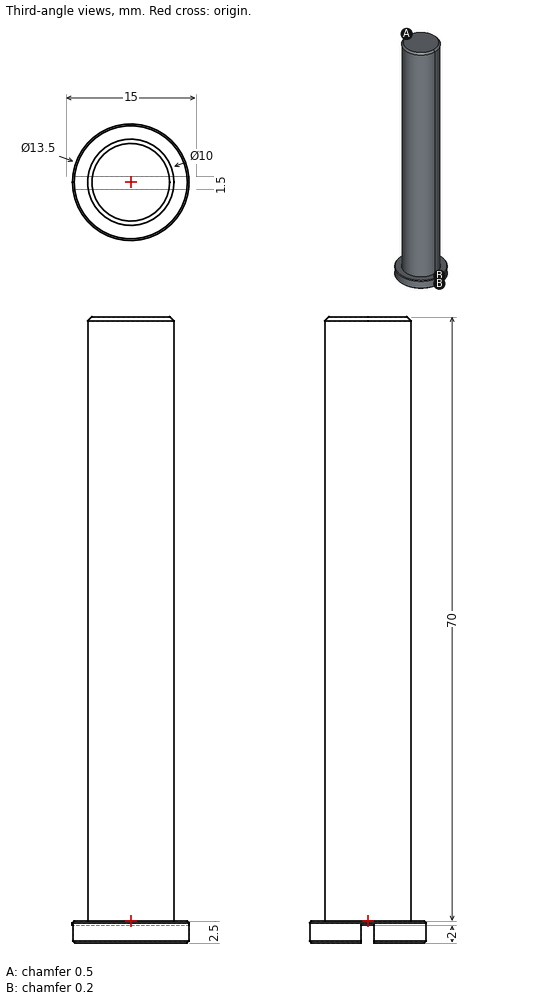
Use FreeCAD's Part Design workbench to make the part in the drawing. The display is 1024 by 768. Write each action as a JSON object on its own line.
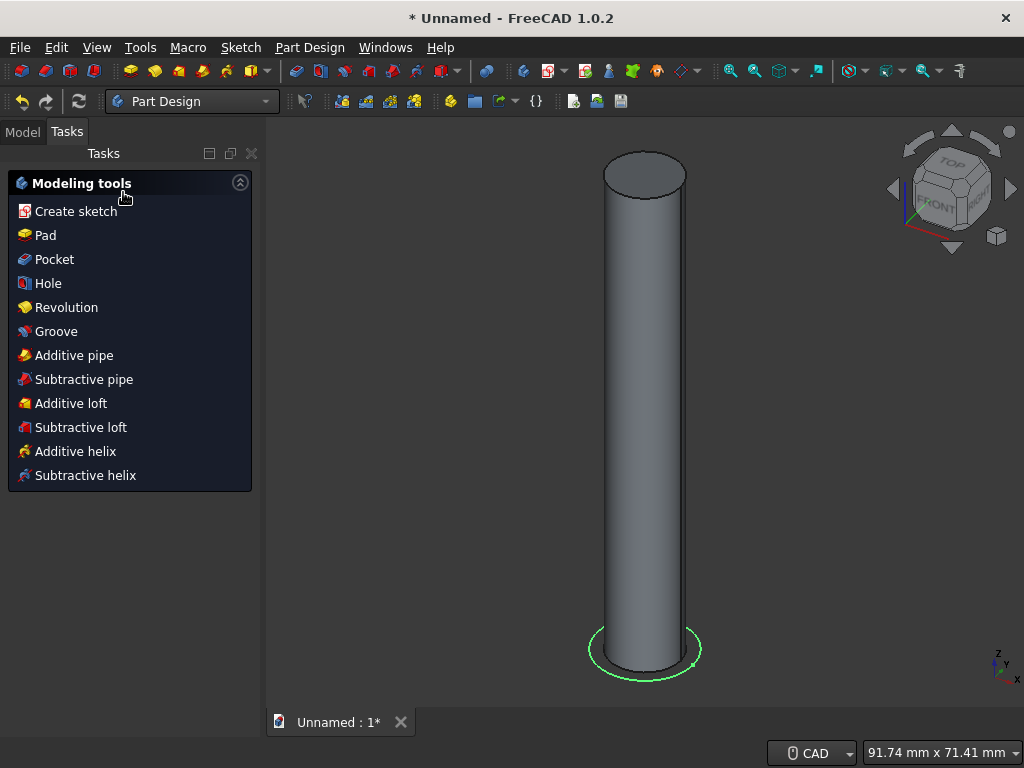
{"action": "left_click", "coordinate": [132, 72]}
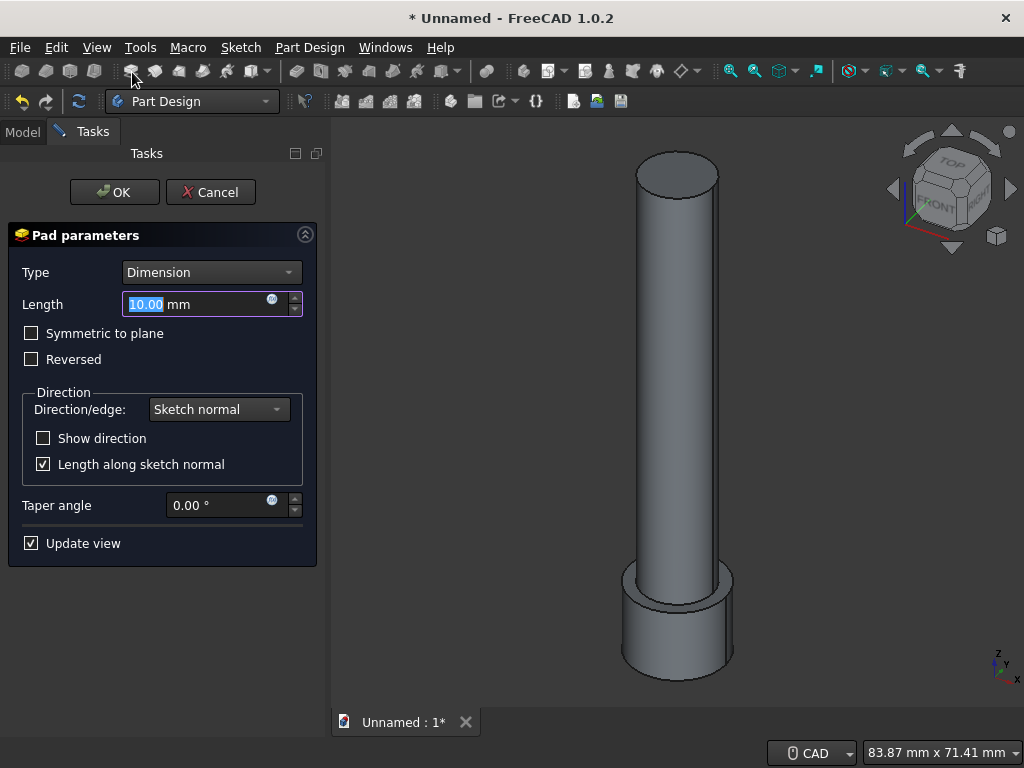
{"action": "type", "text": "2.5"}
{"action": "key", "text": "Tab"}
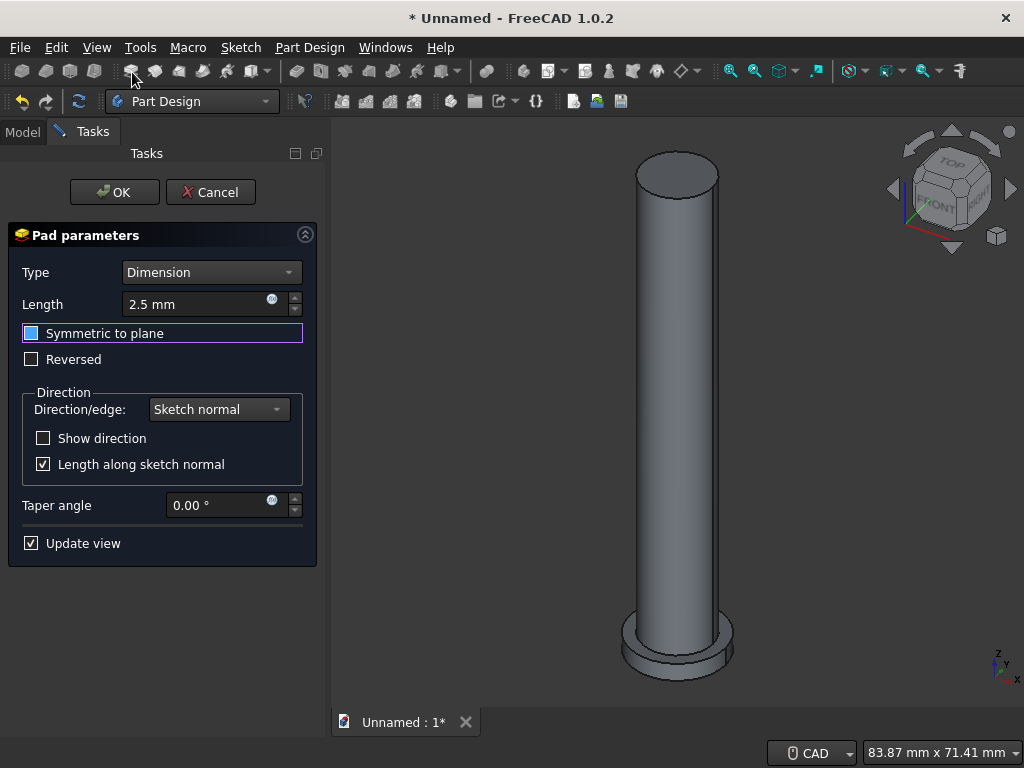
{"action": "left_click", "coordinate": [30, 359]}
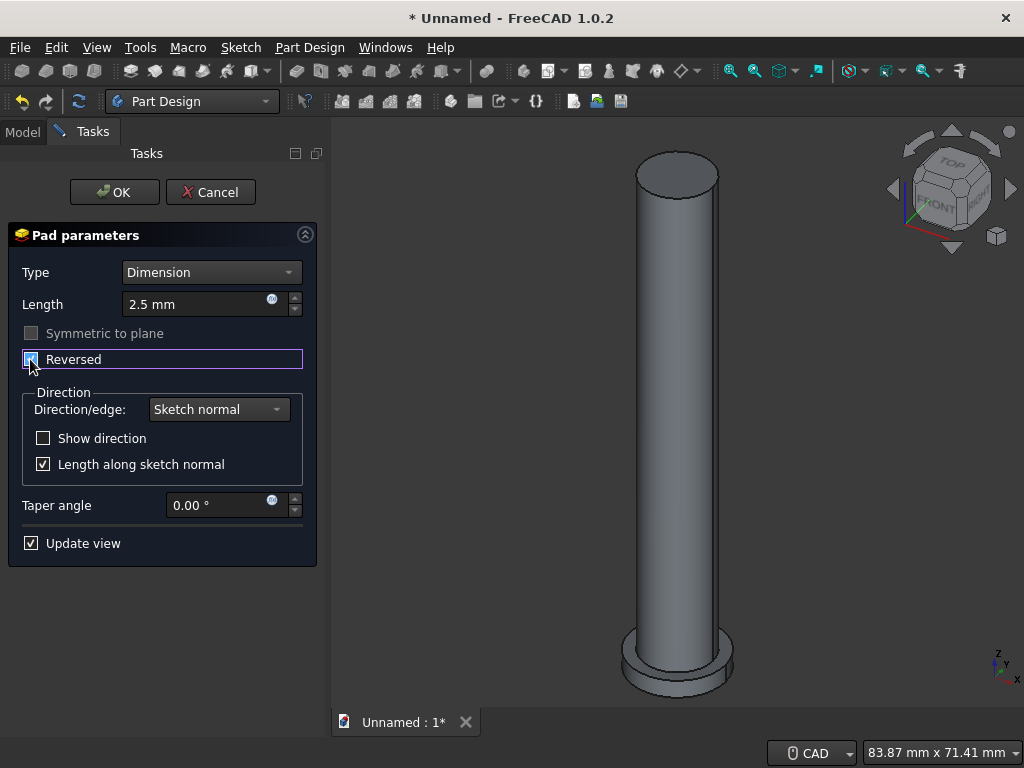
{"action": "left_click", "coordinate": [115, 192]}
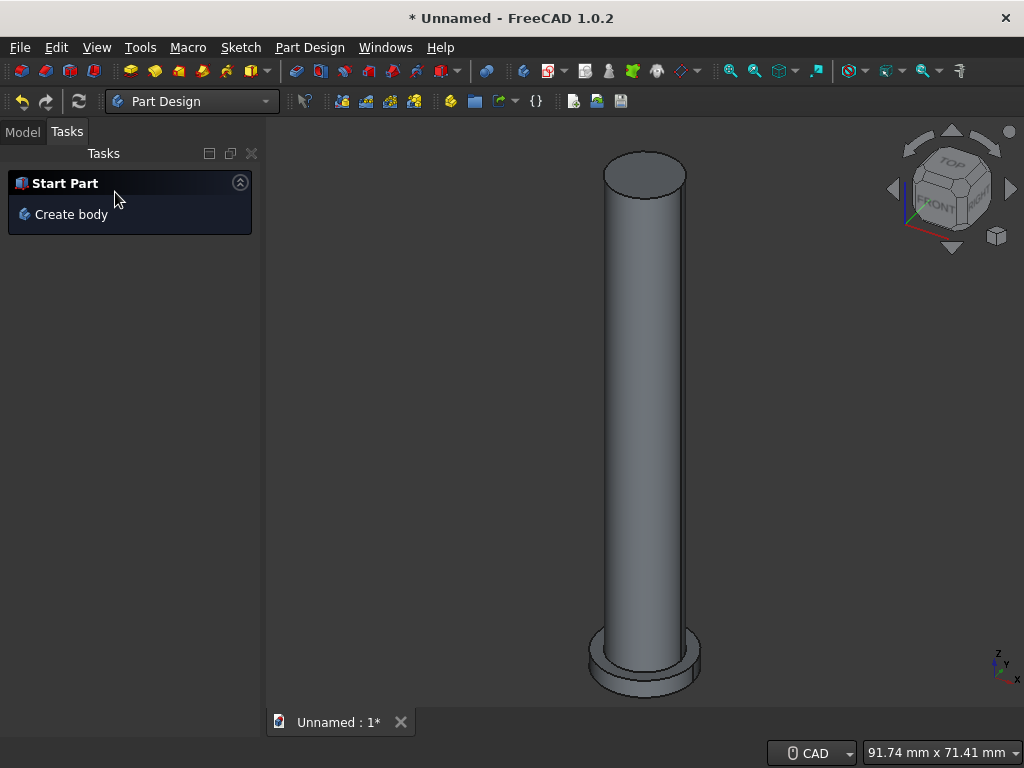
{"action": "left_click", "coordinate": [732, 72]}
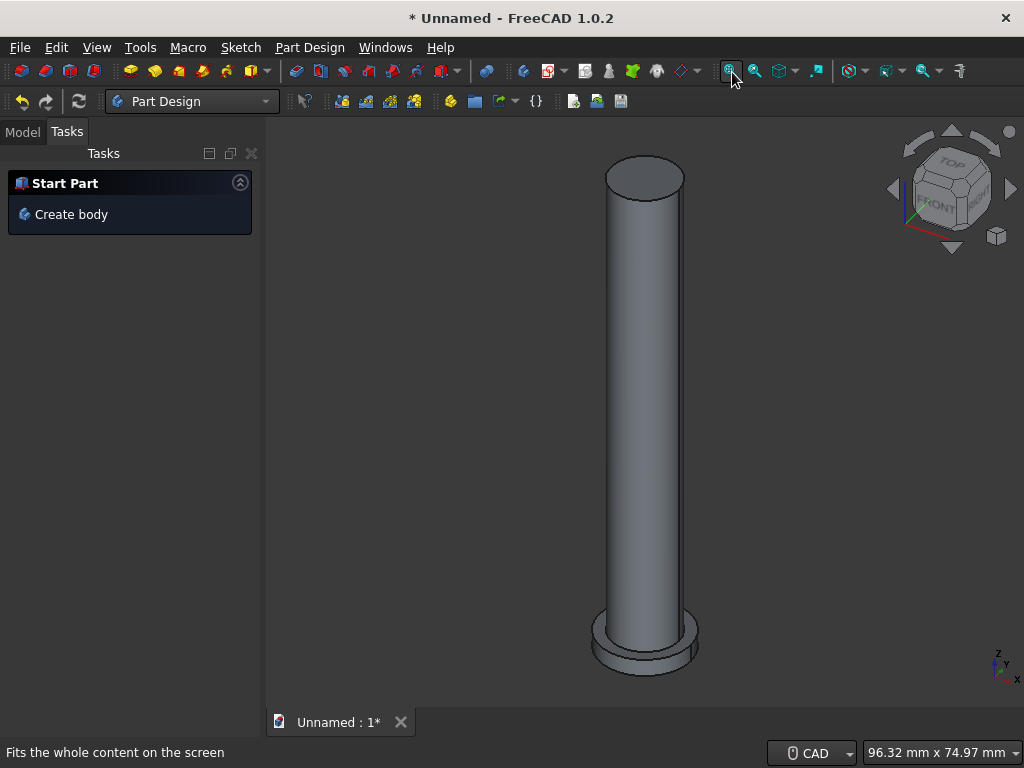
{"action": "left_click", "coordinate": [611, 166]}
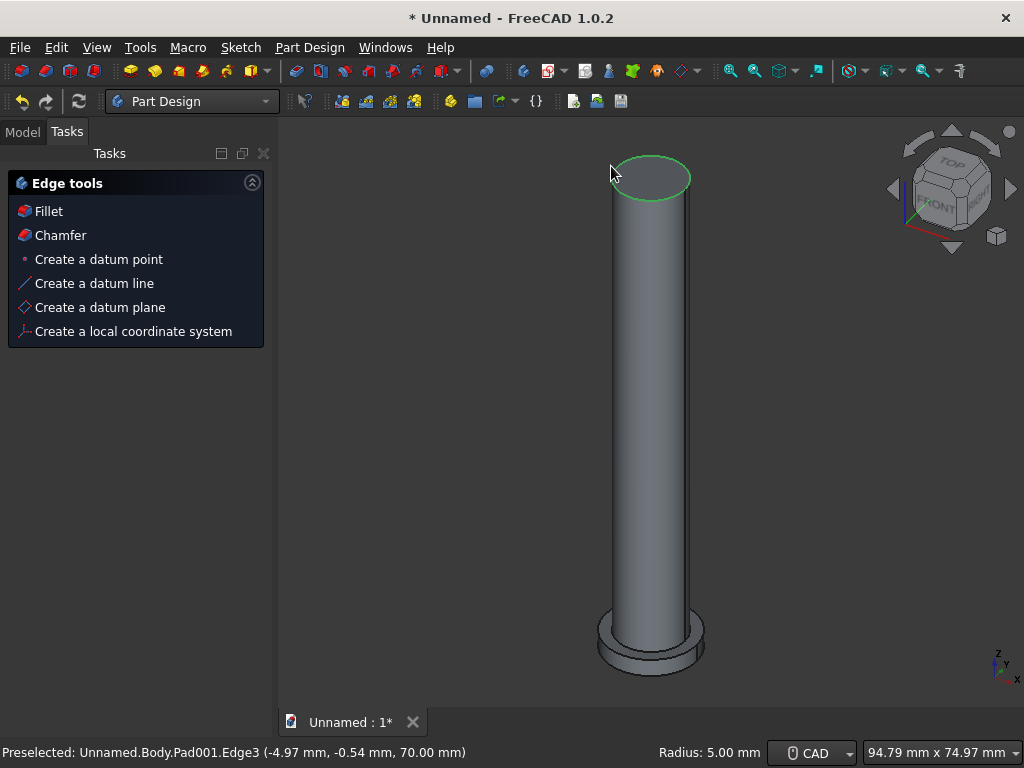
{"action": "left_click", "coordinate": [46, 72]}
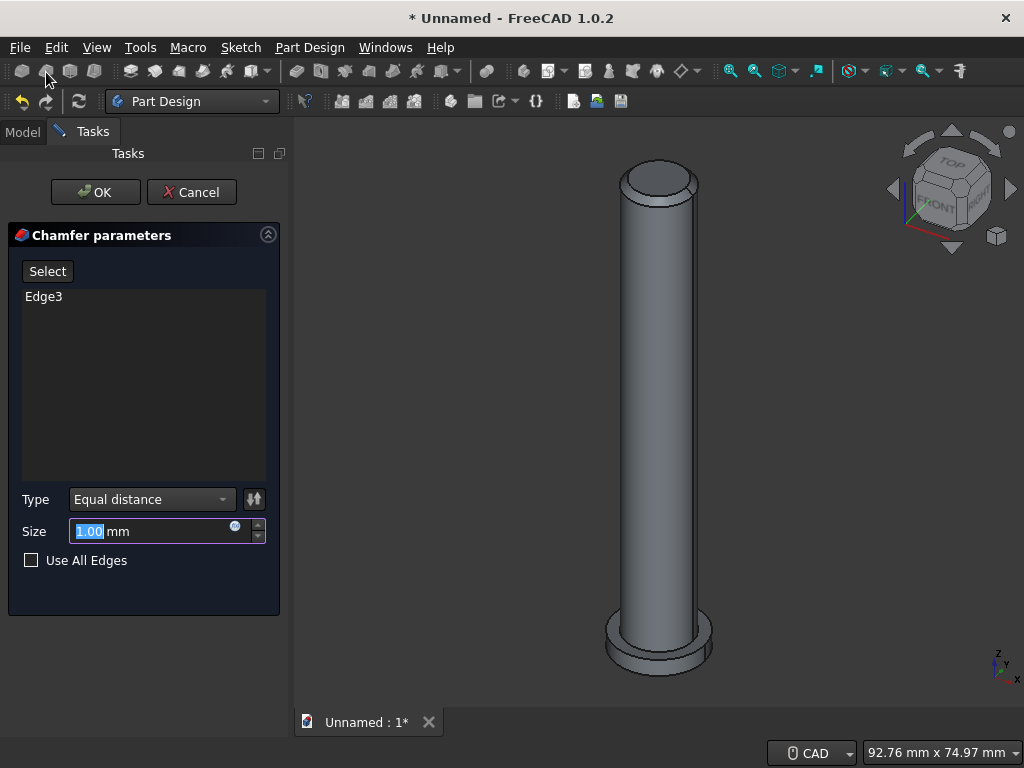
{"action": "type", "text": "0.5"}
{"action": "key", "text": "Tab"}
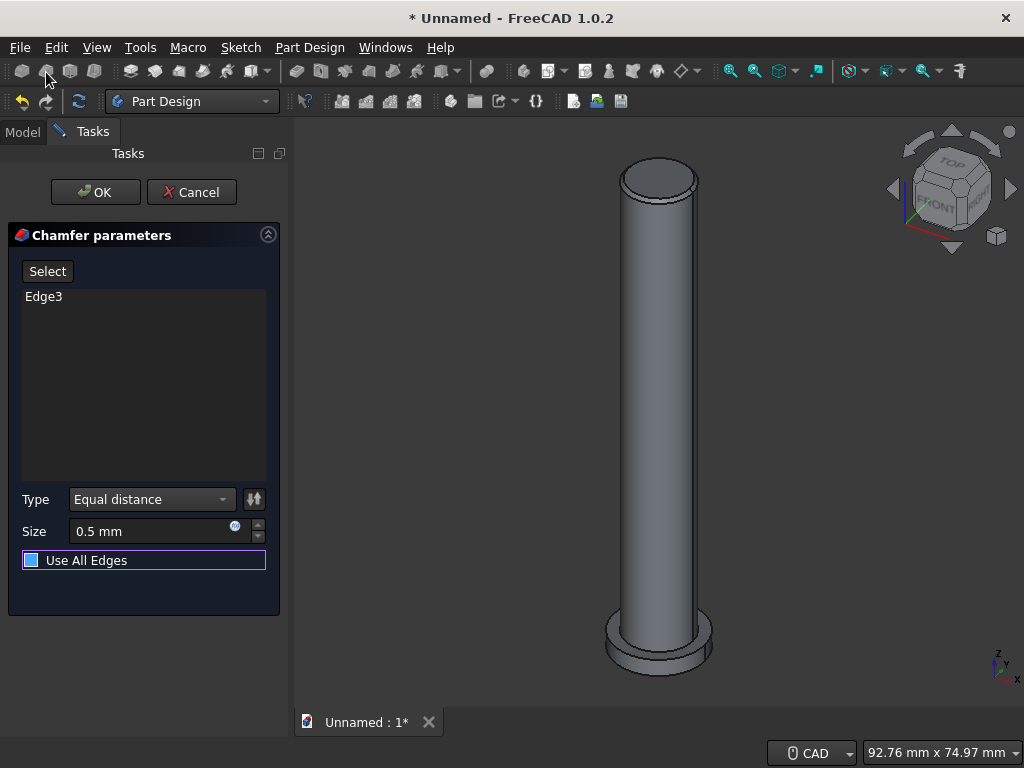
{"action": "left_click", "coordinate": [96, 192]}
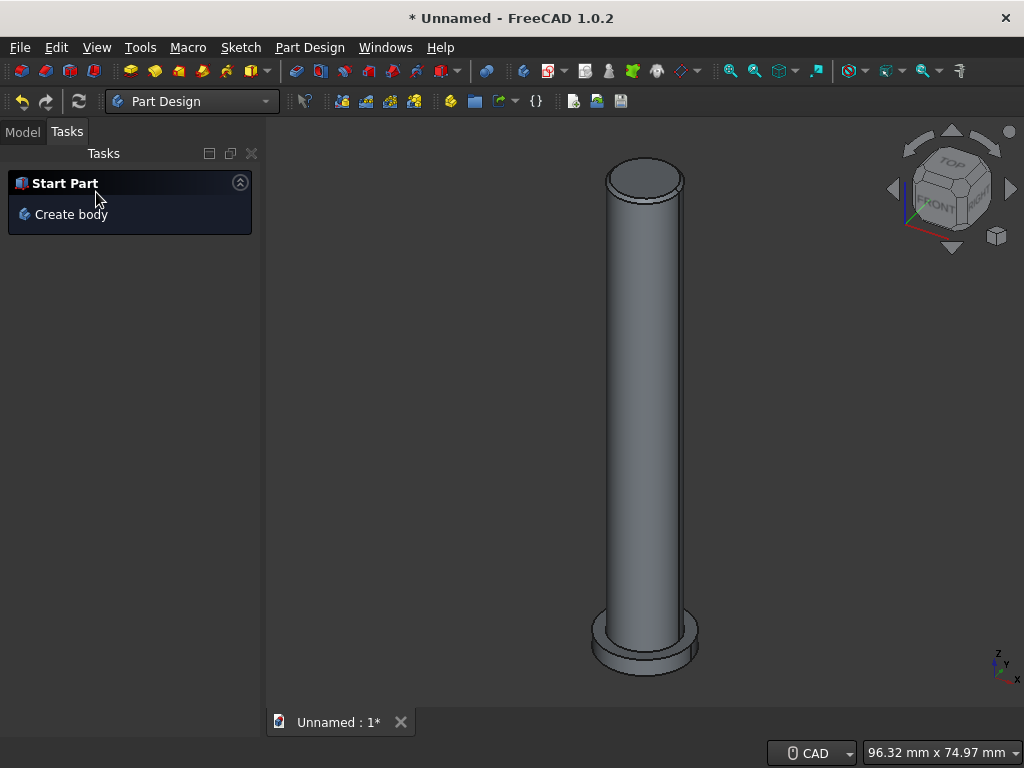
{"action": "left_click", "coordinate": [592, 632]}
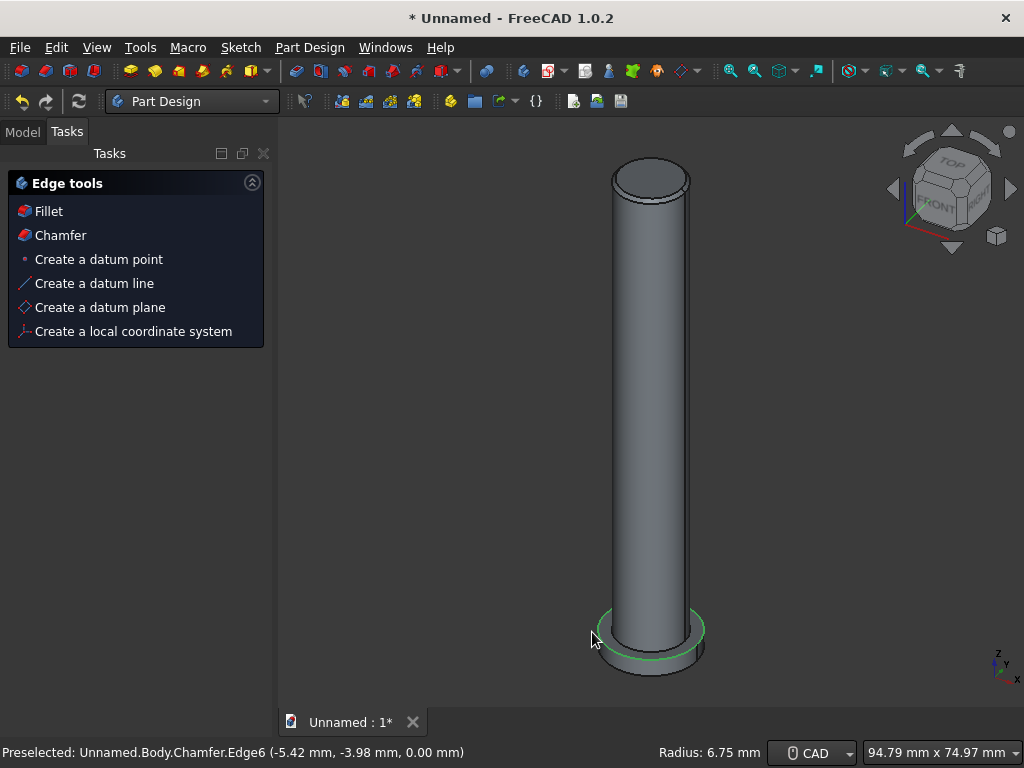
{"action": "key", "text": "0"}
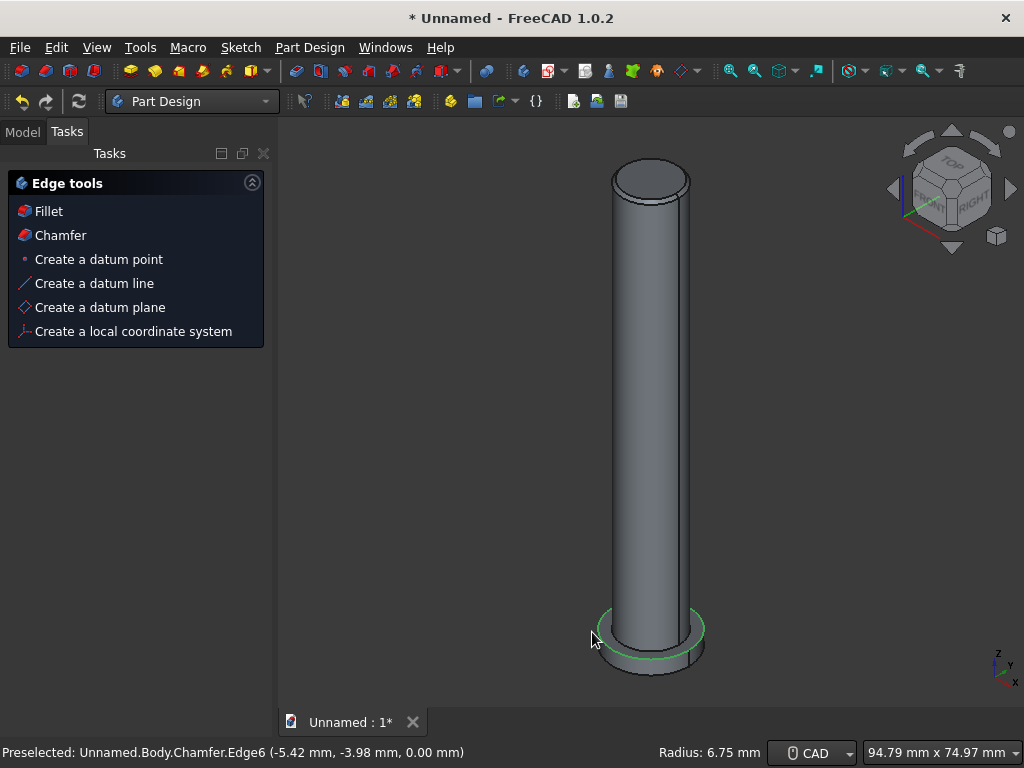
{"action": "key", "text": "2"}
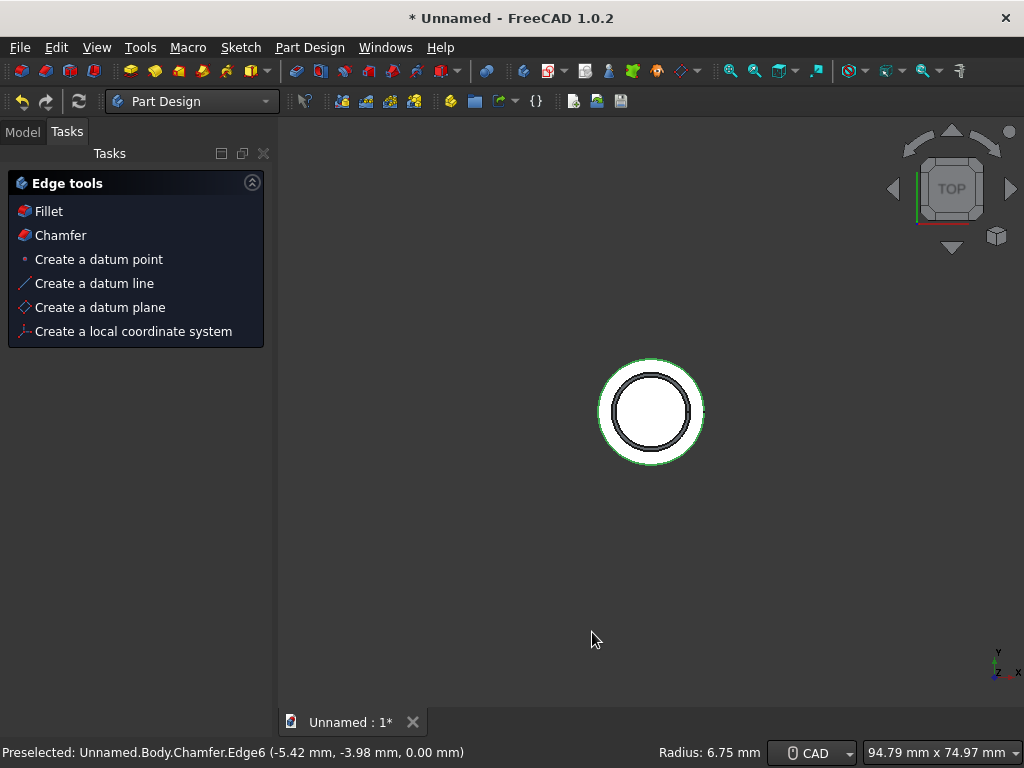
{"action": "left_click", "coordinate": [732, 72]}